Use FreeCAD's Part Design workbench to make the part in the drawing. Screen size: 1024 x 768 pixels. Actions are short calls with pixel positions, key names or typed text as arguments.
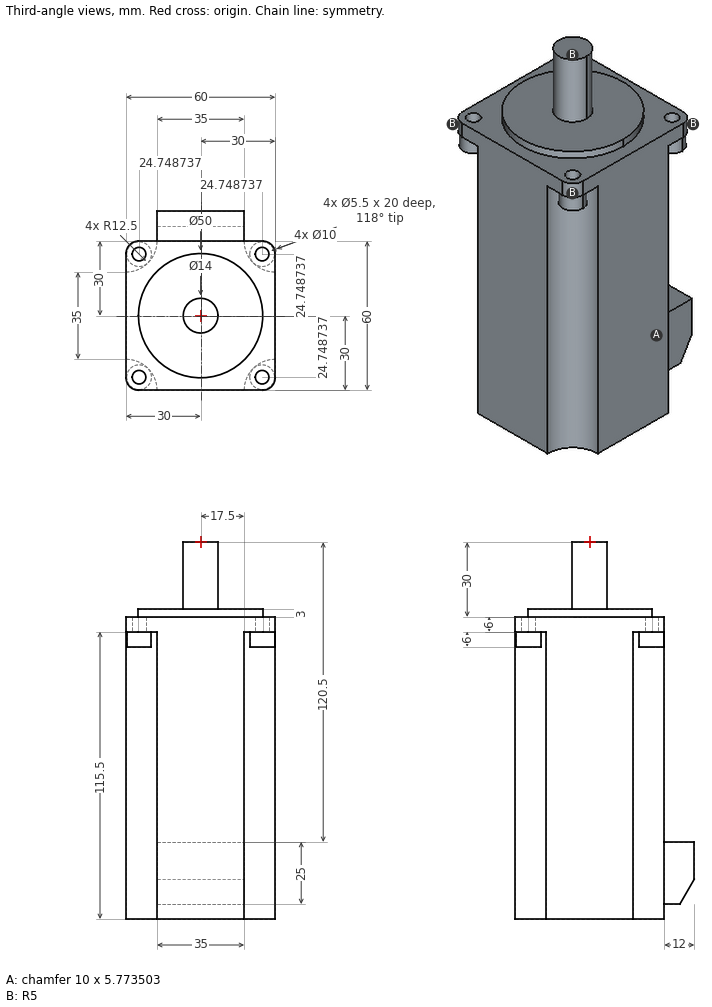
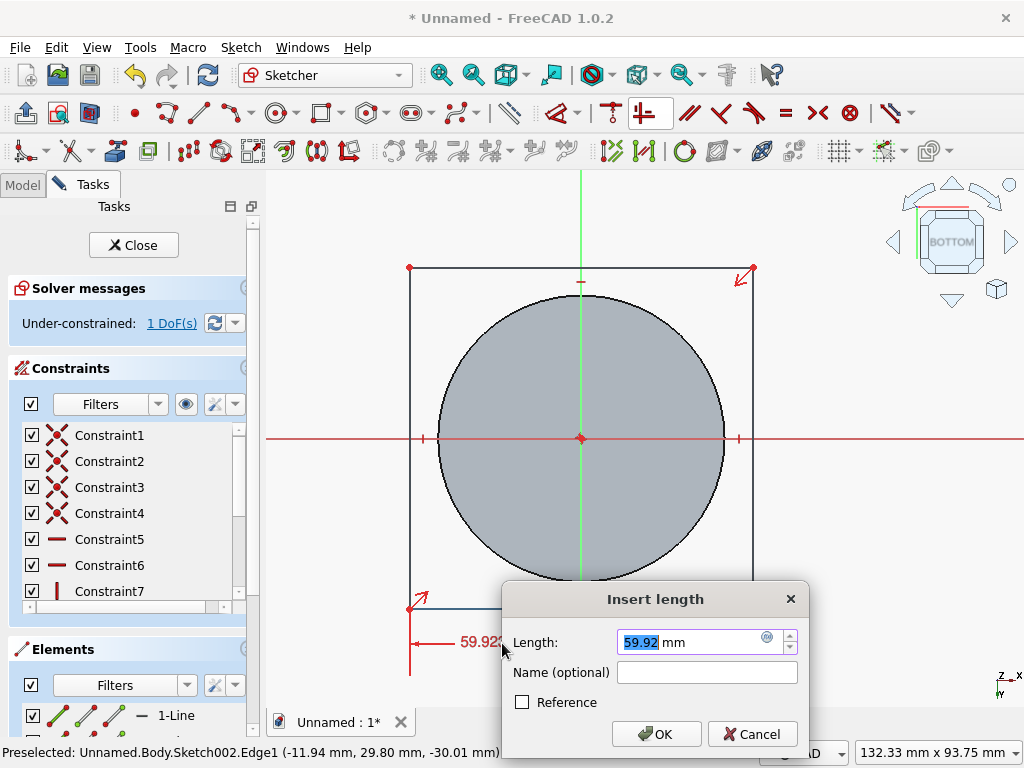
text(60)
key(Return)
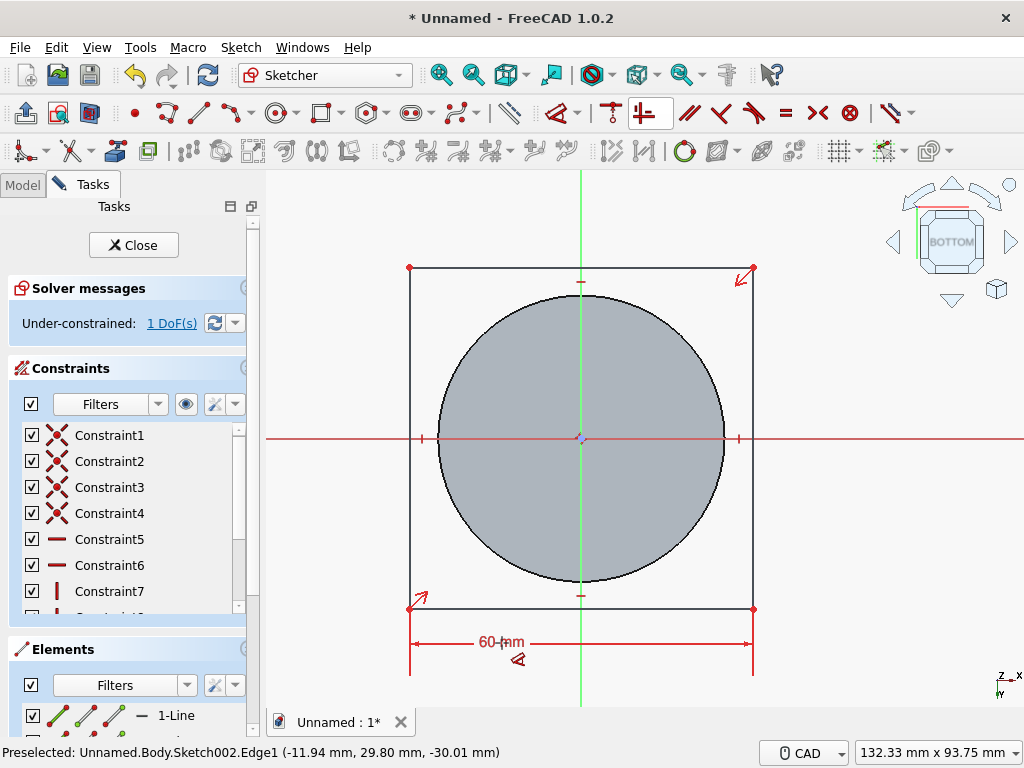
click(753, 507)
click(787, 360)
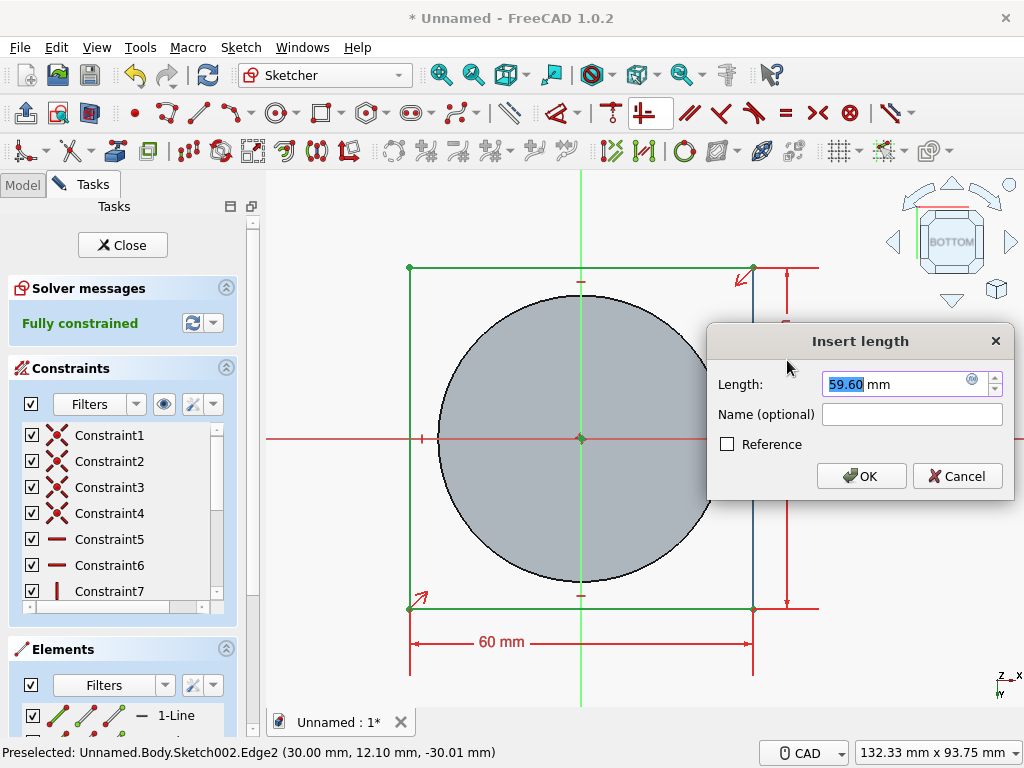
text(60)
key(Return)
key(Escape)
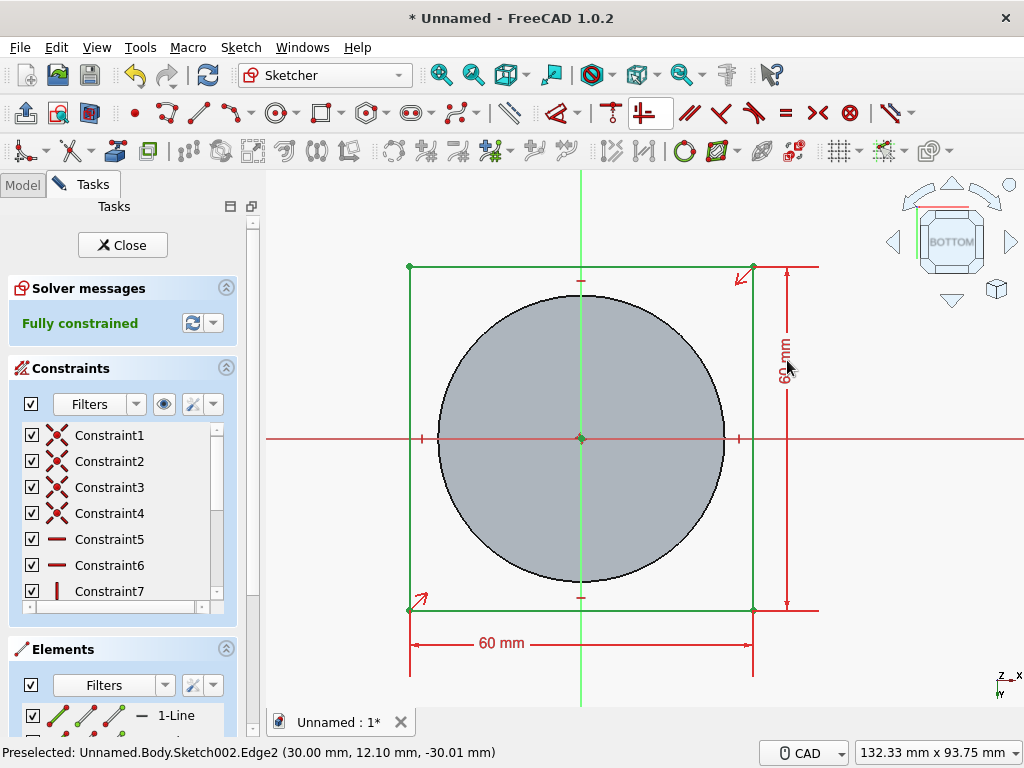
click(123, 245)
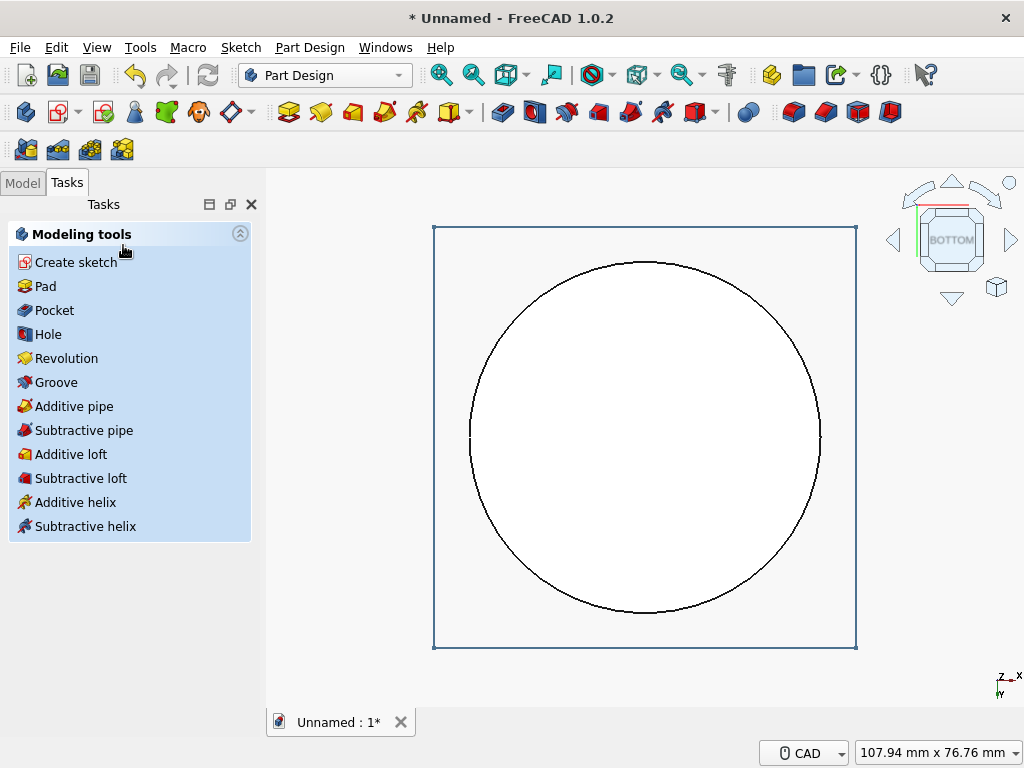
click(290, 112)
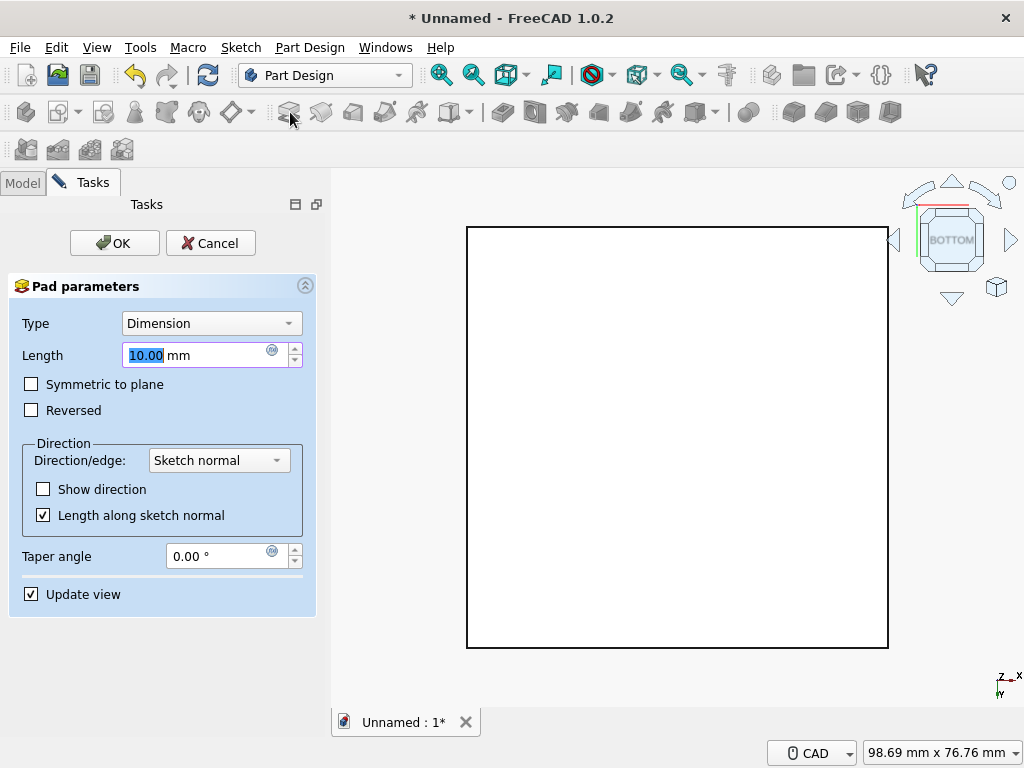
text(6)
key(Tab)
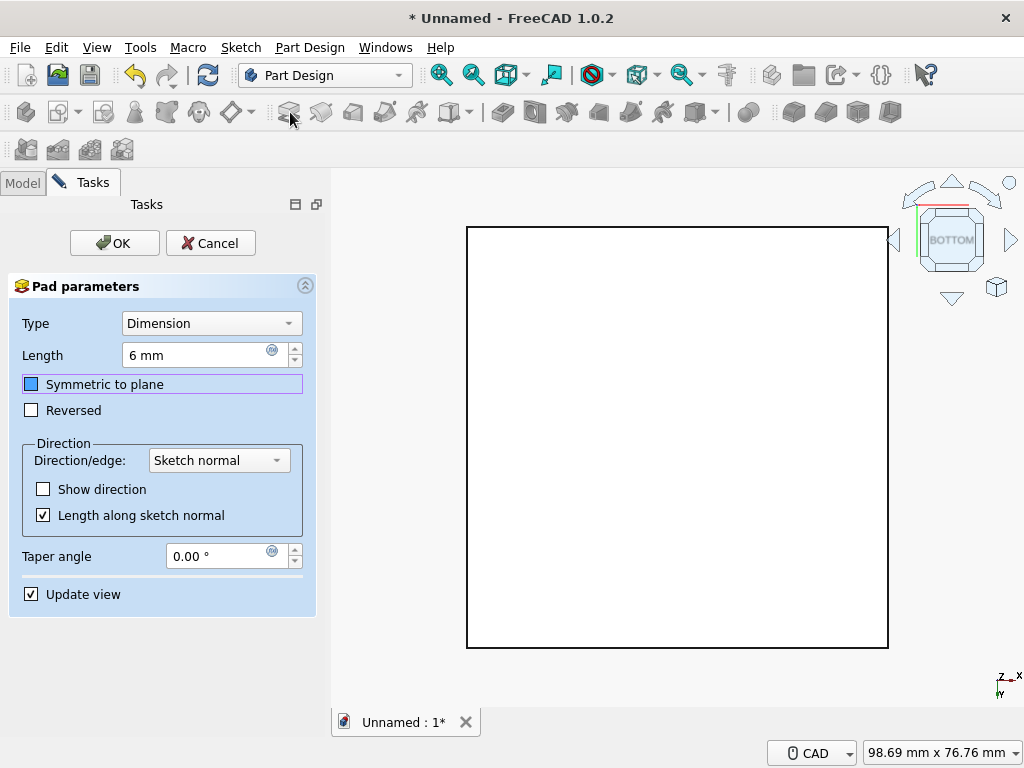
click(115, 243)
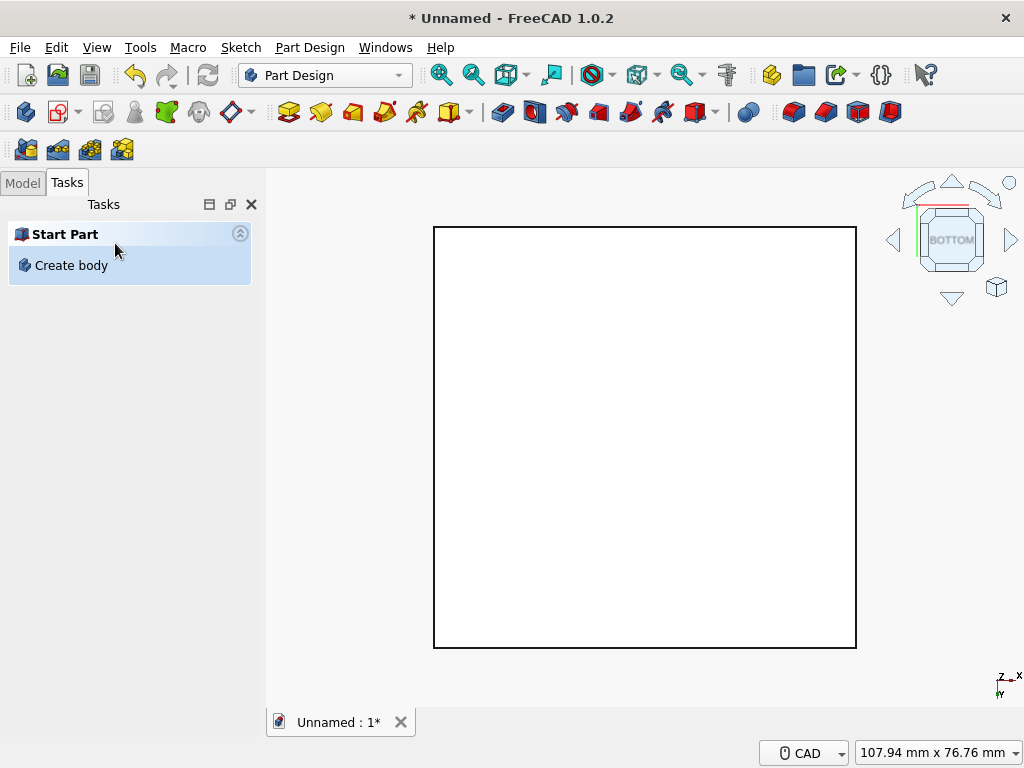
click(645, 436)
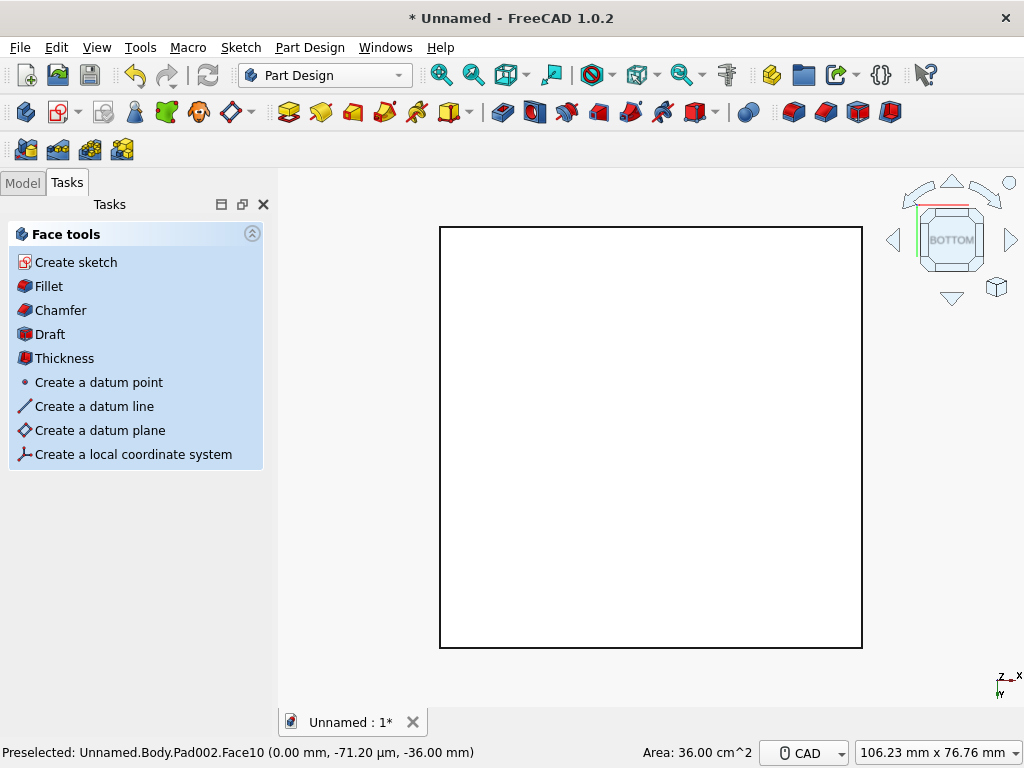
click(58, 112)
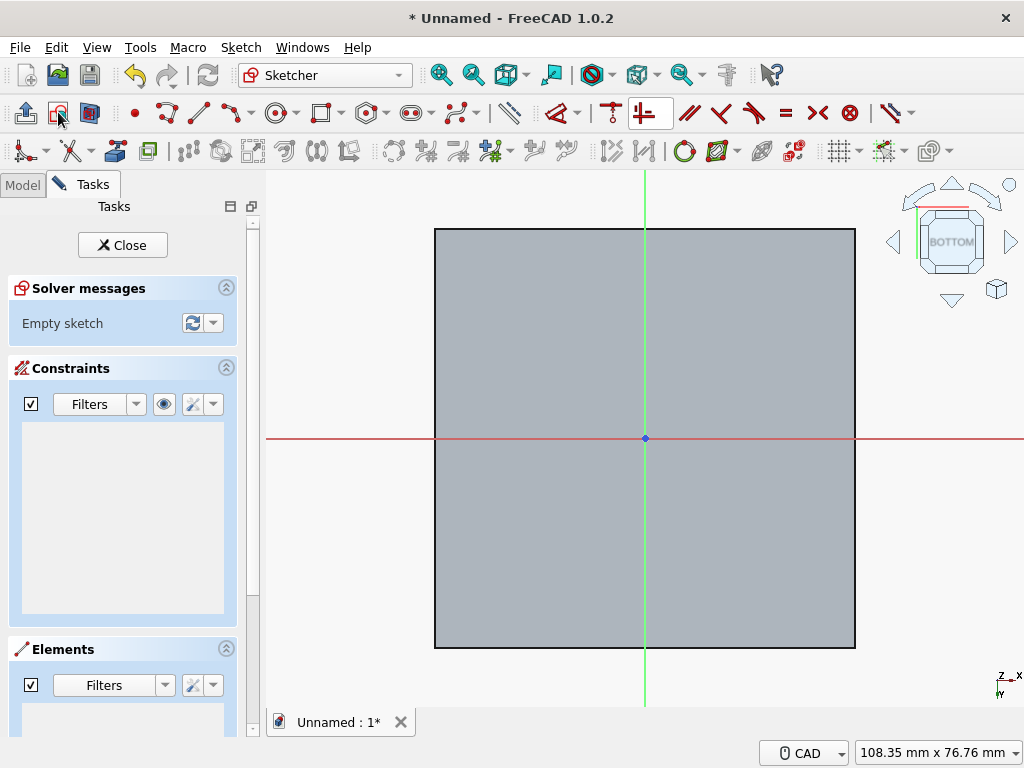
scroll(294, 439, down, 1)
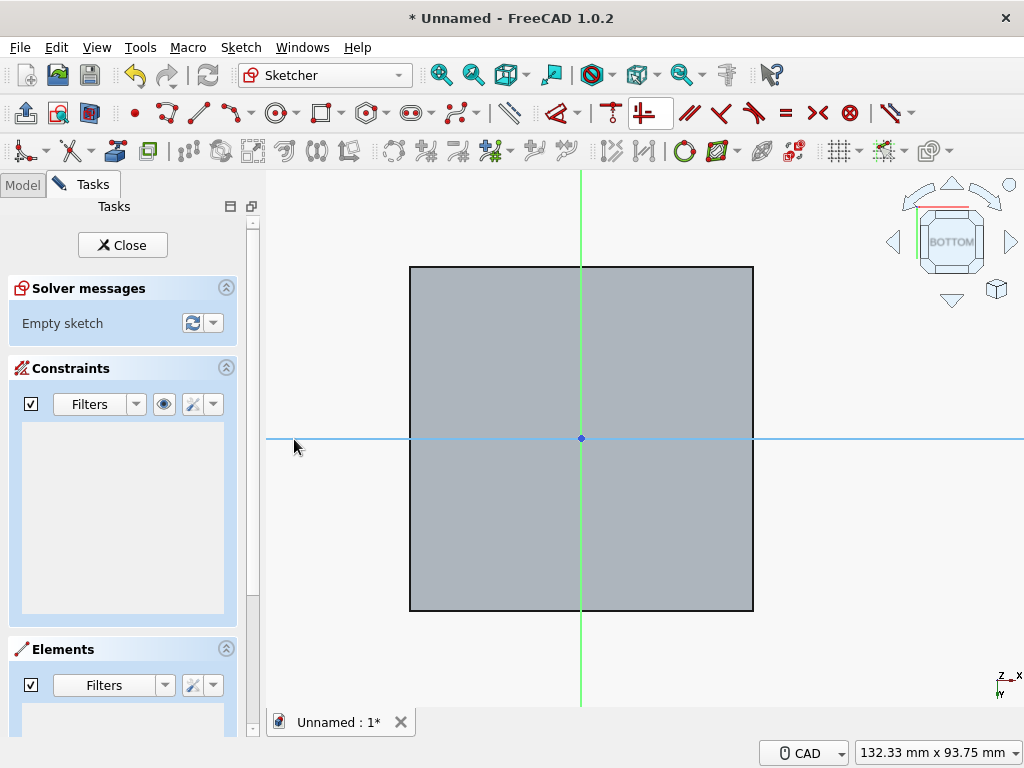
click(200, 114)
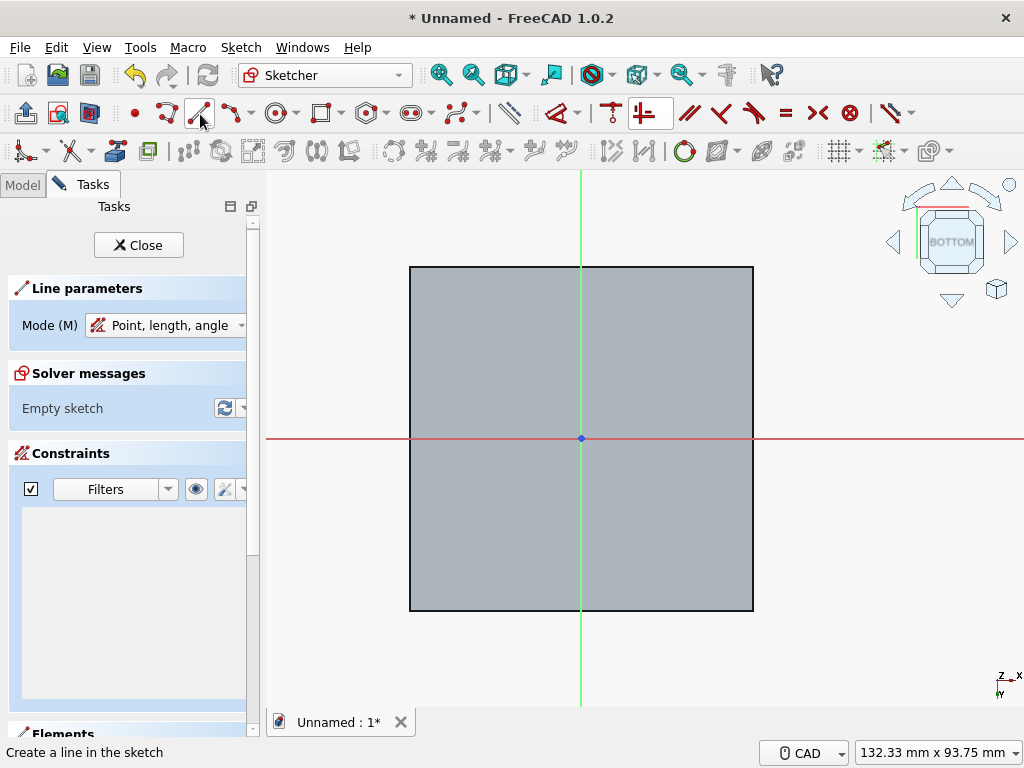
click(410, 338)
click(410, 539)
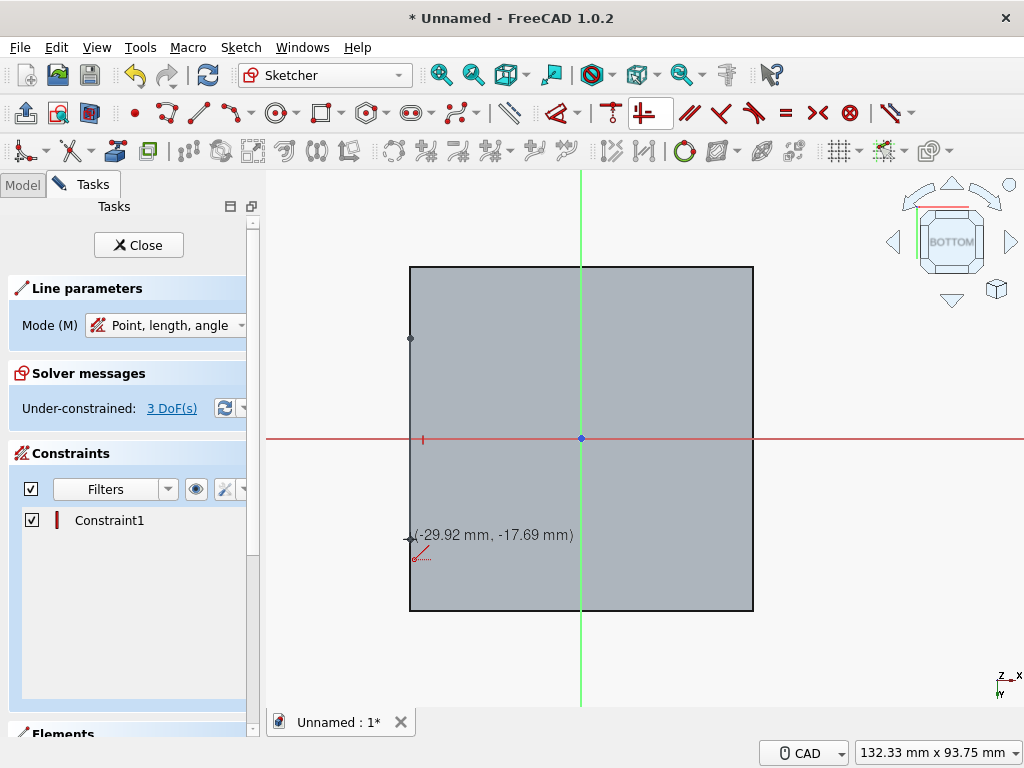
click(481, 611)
click(682, 611)